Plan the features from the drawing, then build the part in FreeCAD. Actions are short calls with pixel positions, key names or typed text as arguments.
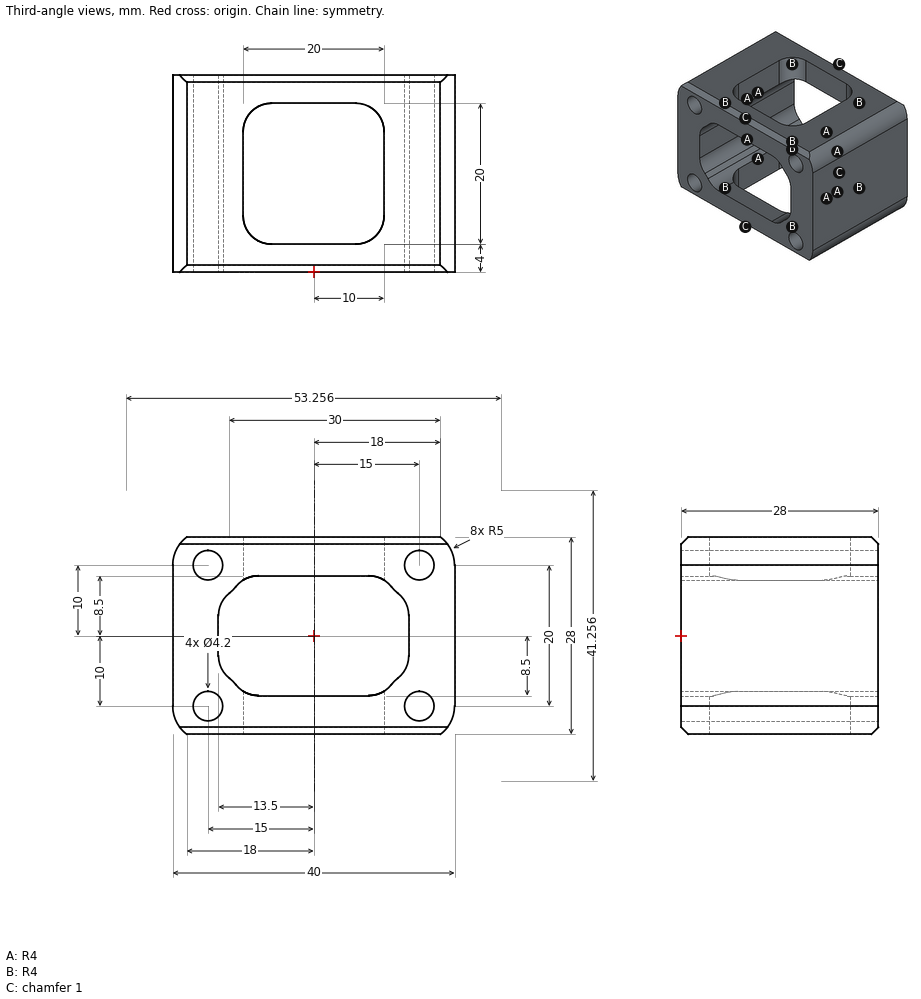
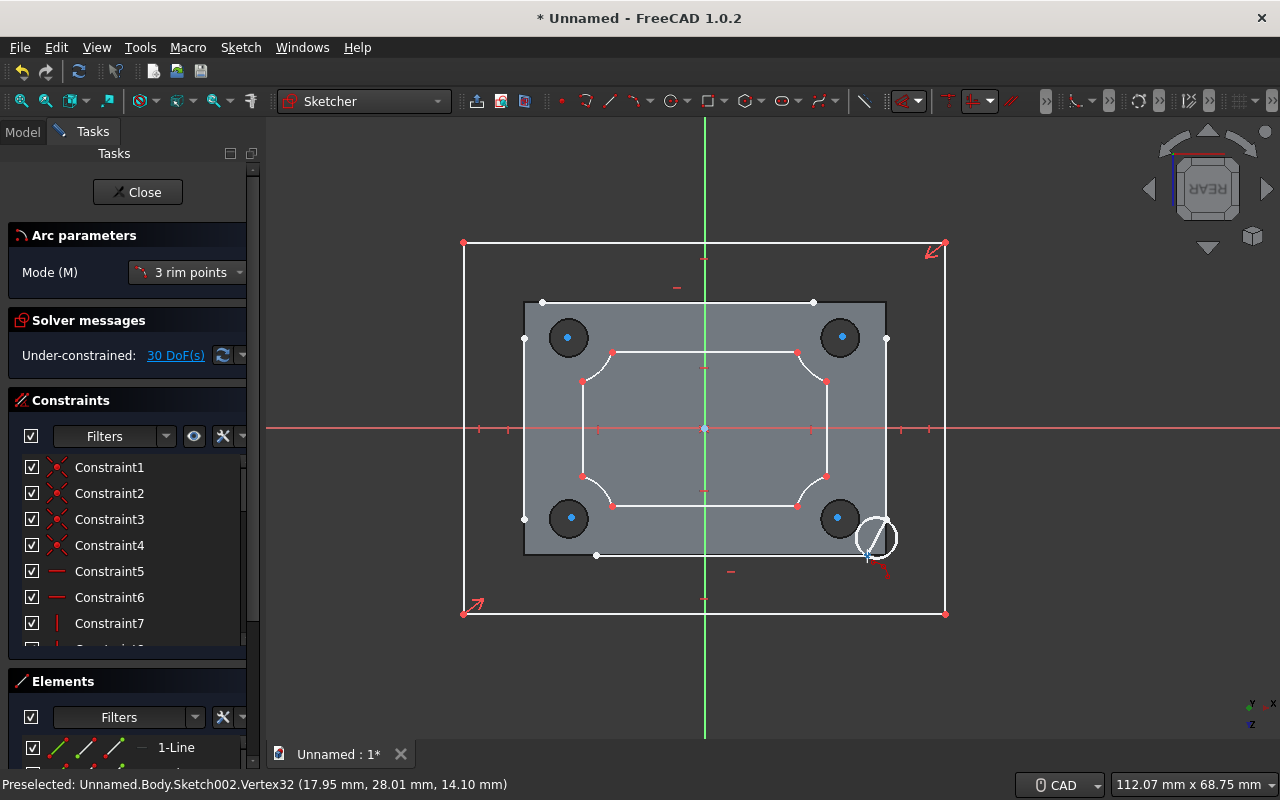
scroll(881, 539, up, 7)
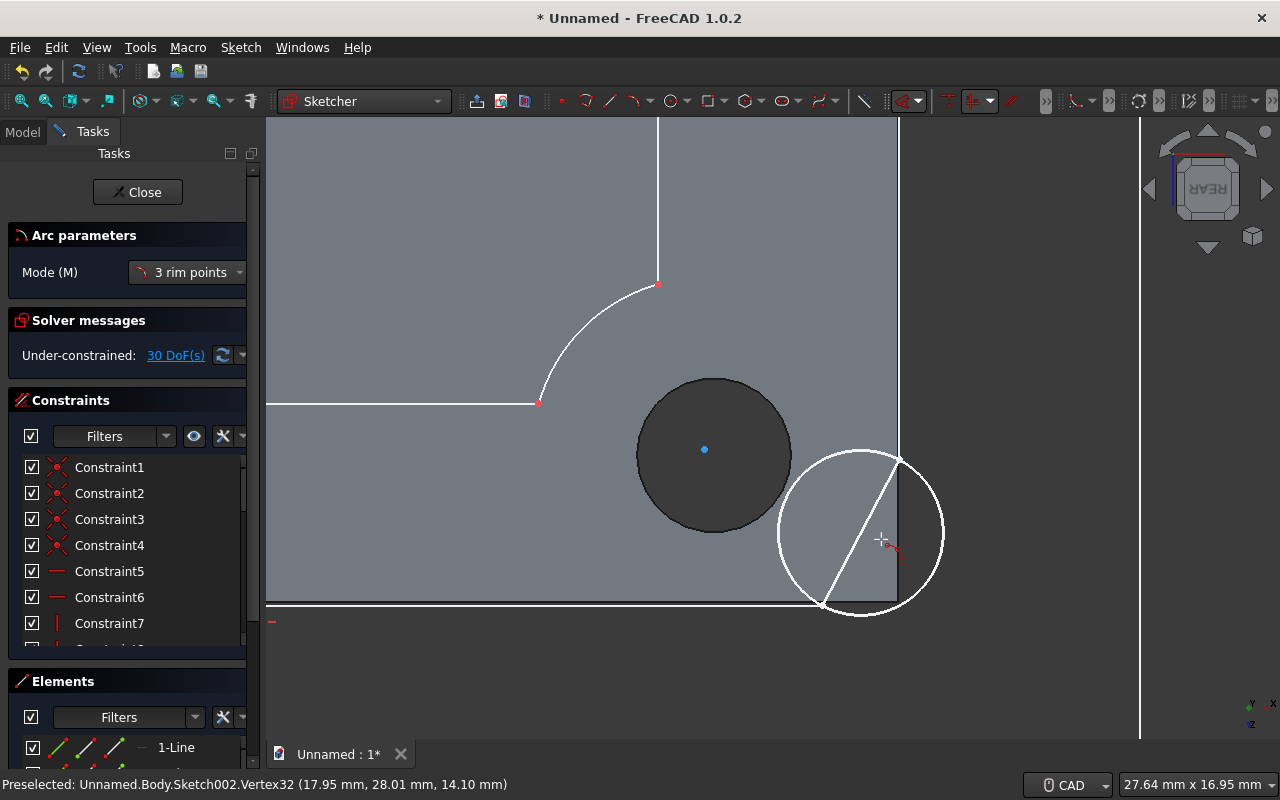
click(878, 537)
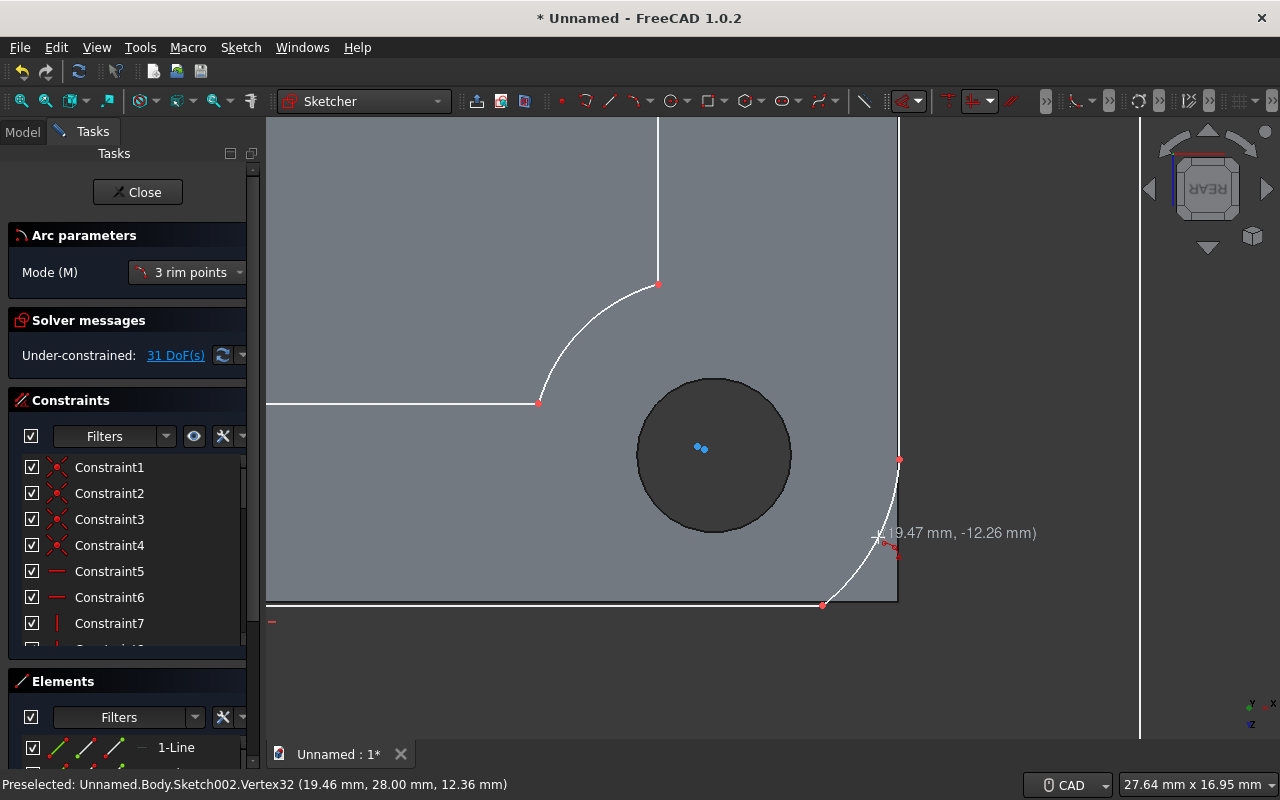
scroll(882, 539, down, 7)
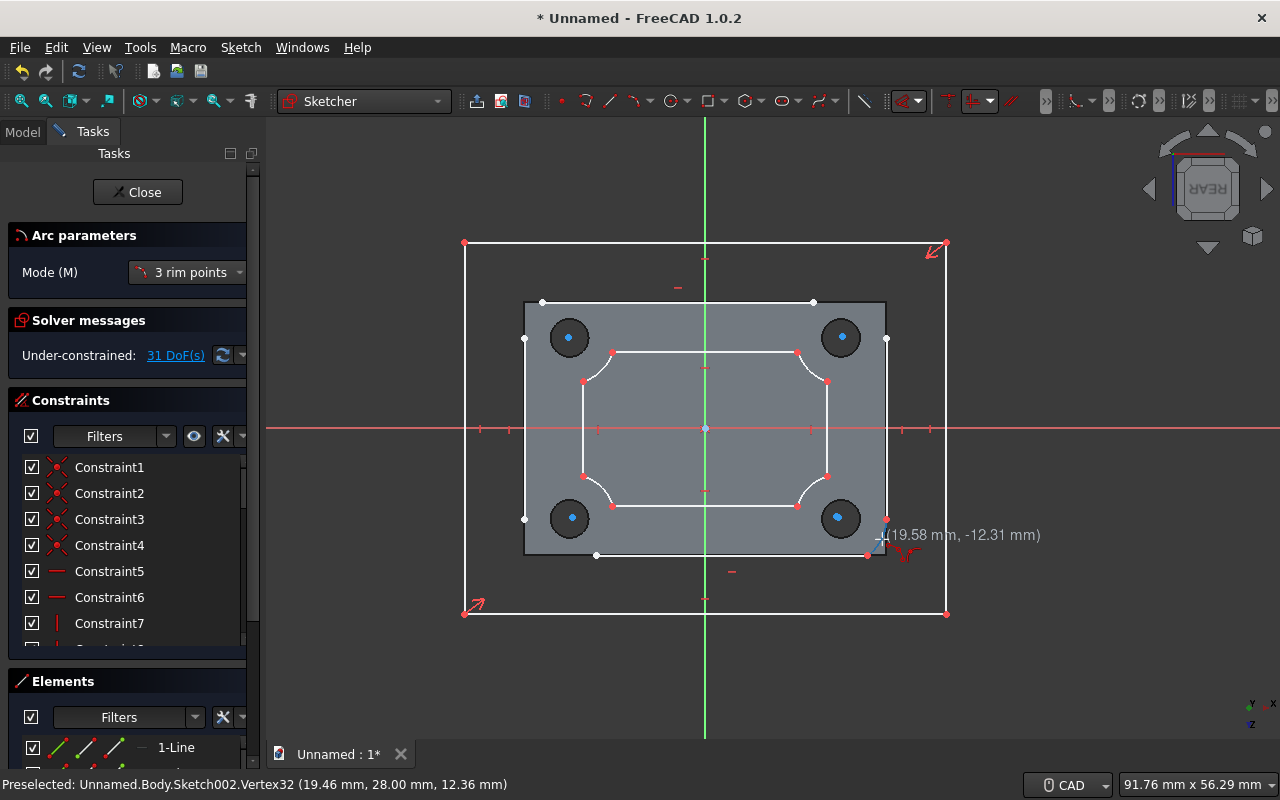
click(597, 556)
click(525, 520)
click(549, 559)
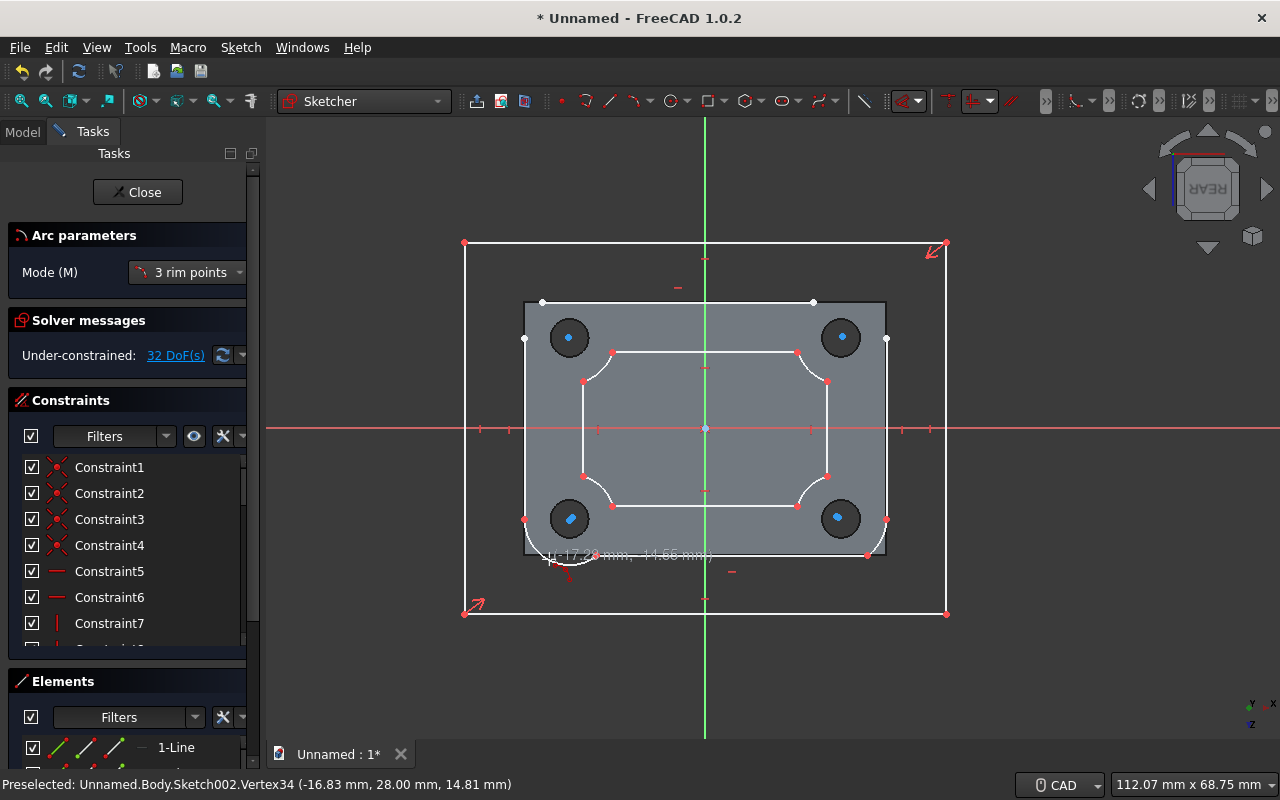
click(525, 339)
click(543, 303)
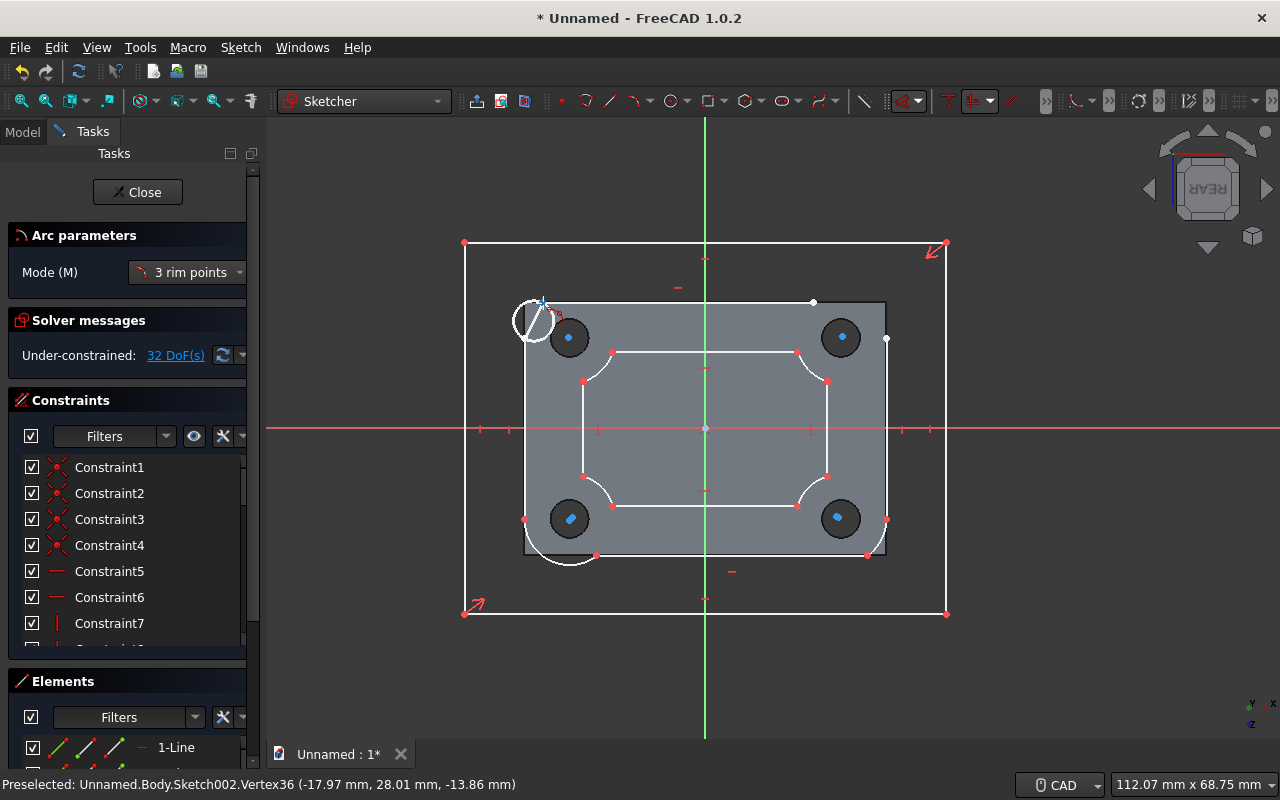
scroll(529, 318, up, 7)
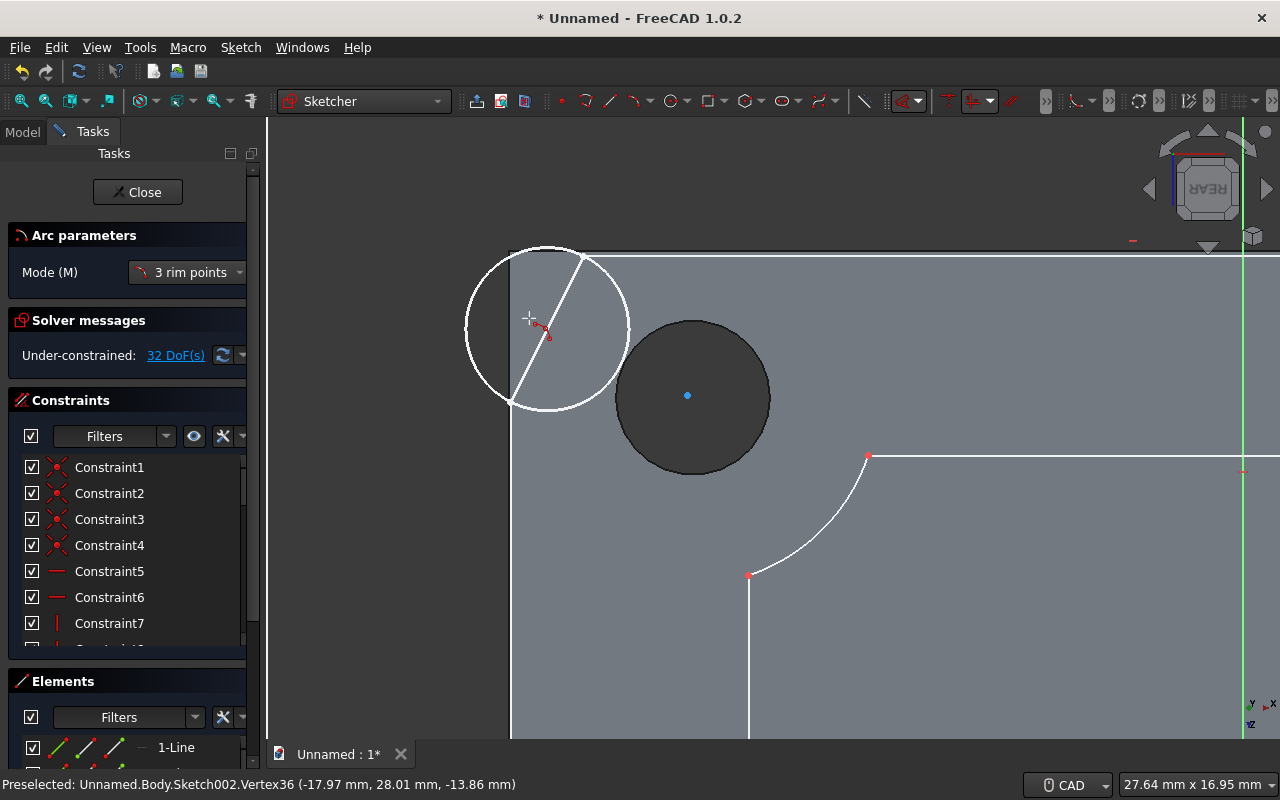
click(529, 316)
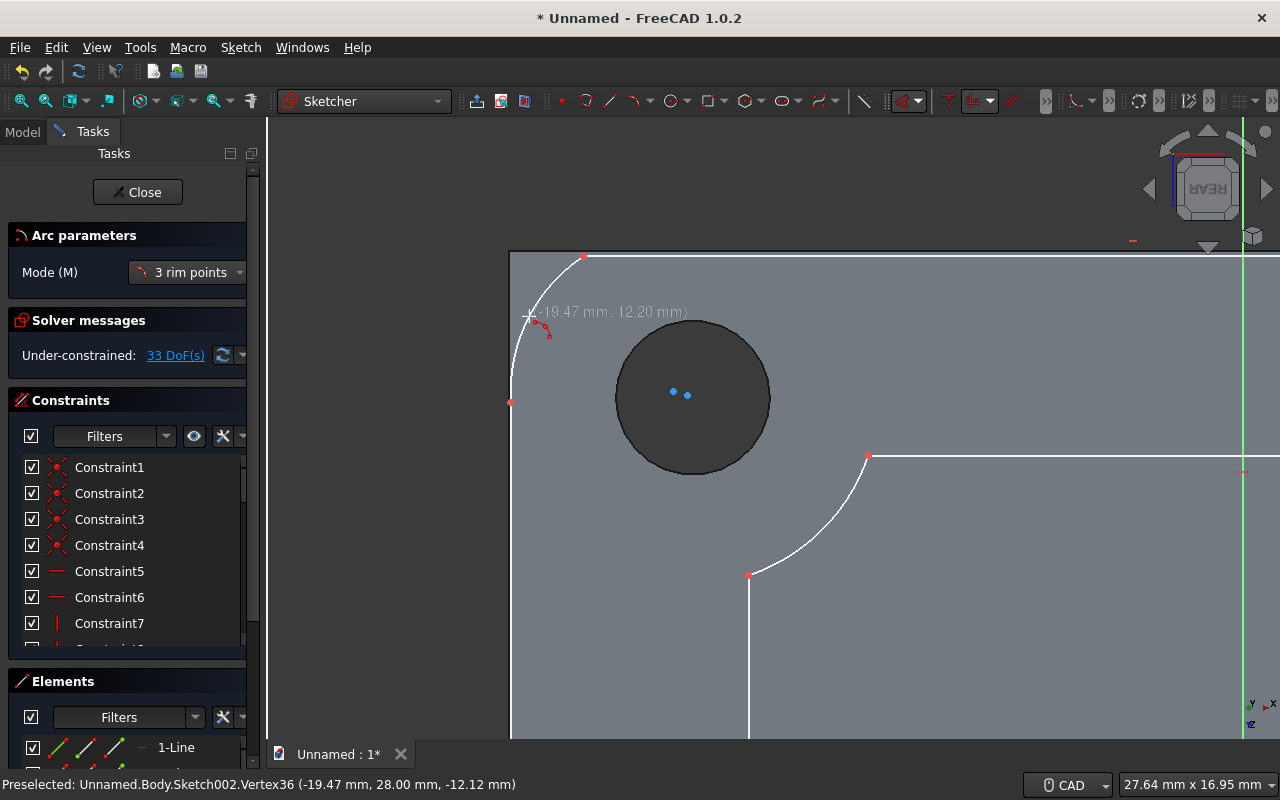
scroll(528, 318, down, 7)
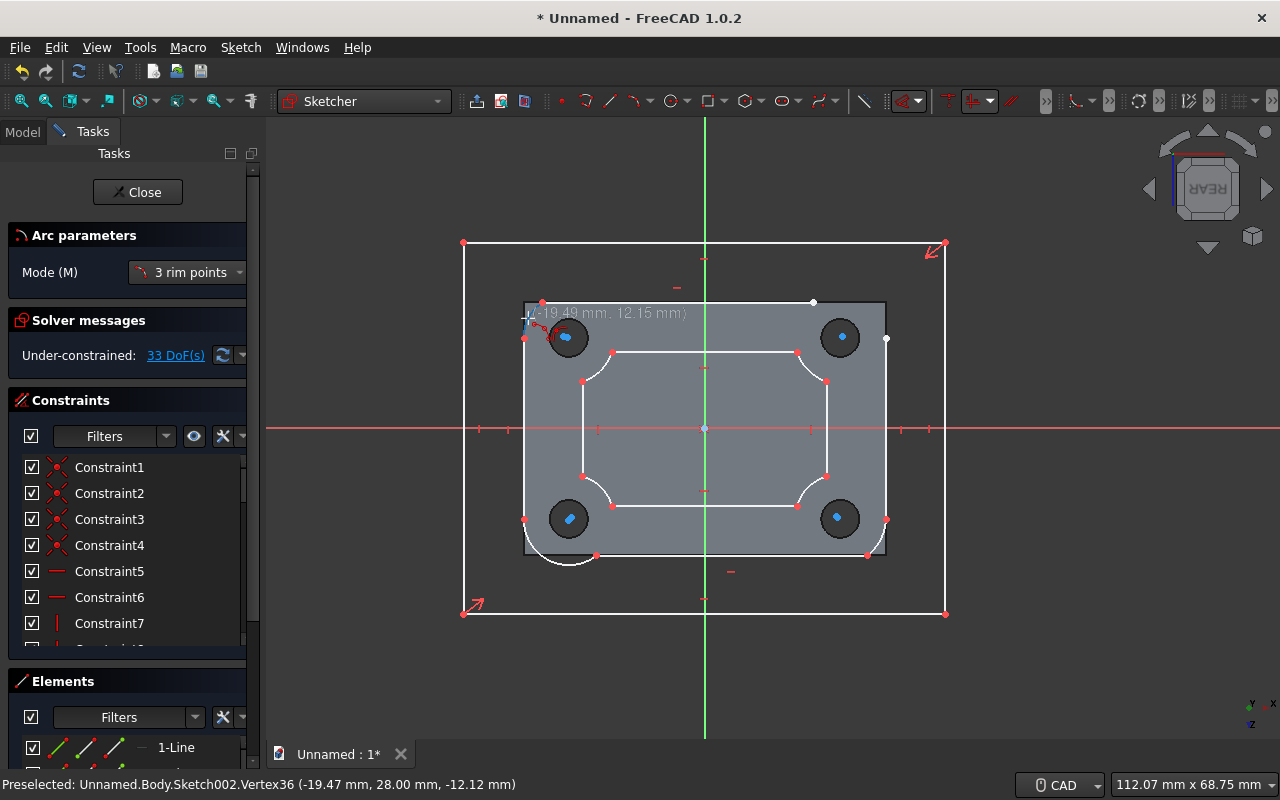
click(813, 303)
click(886, 339)
click(861, 297)
key(Escape)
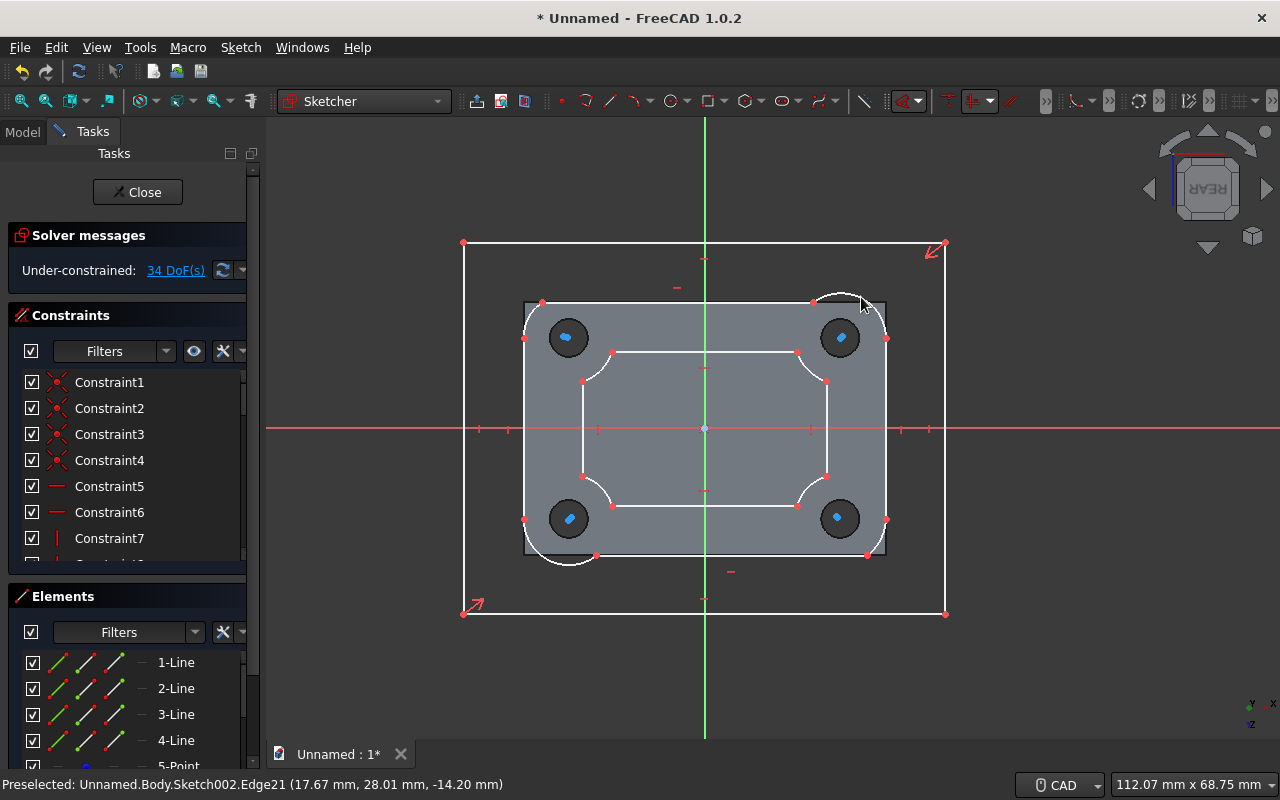
click(886, 393)